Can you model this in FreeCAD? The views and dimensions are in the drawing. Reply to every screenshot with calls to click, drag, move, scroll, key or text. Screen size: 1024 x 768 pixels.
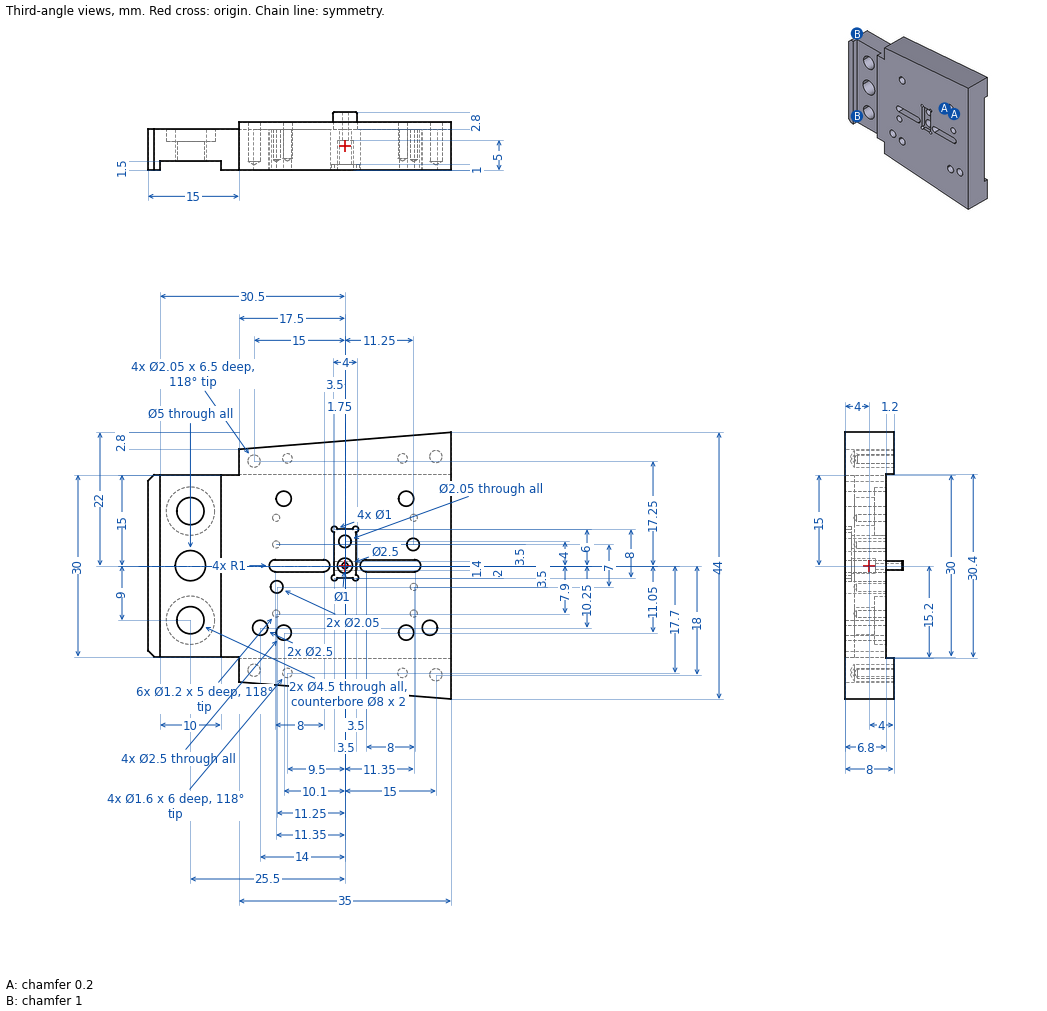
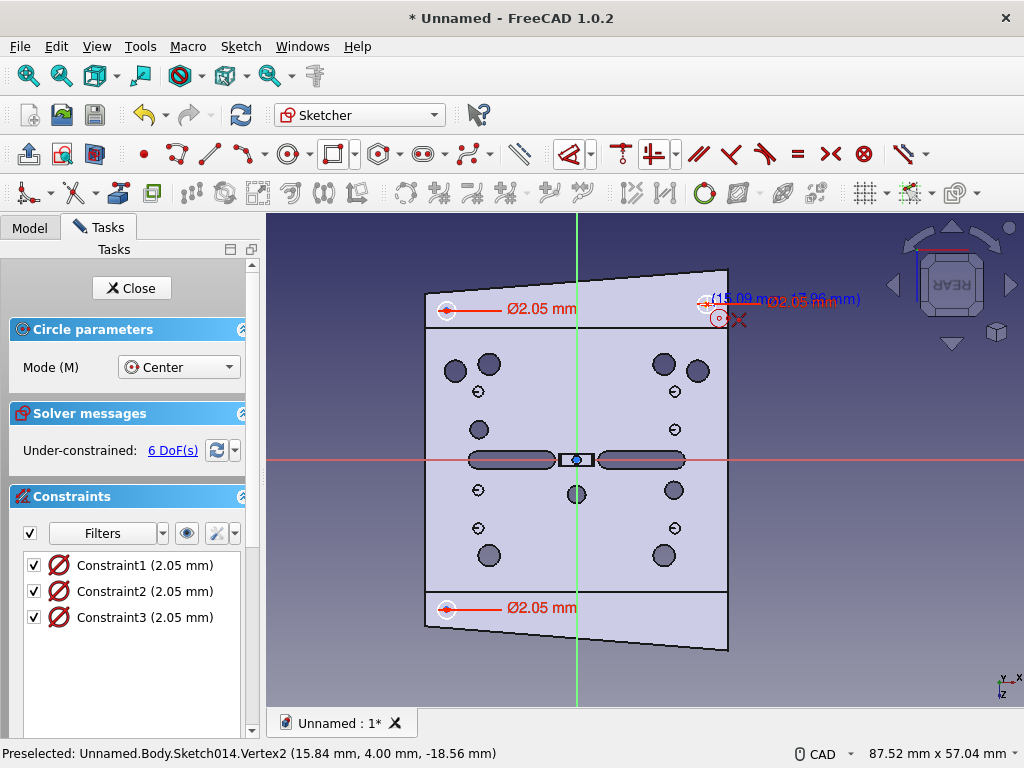
scroll(707, 616, up, 5)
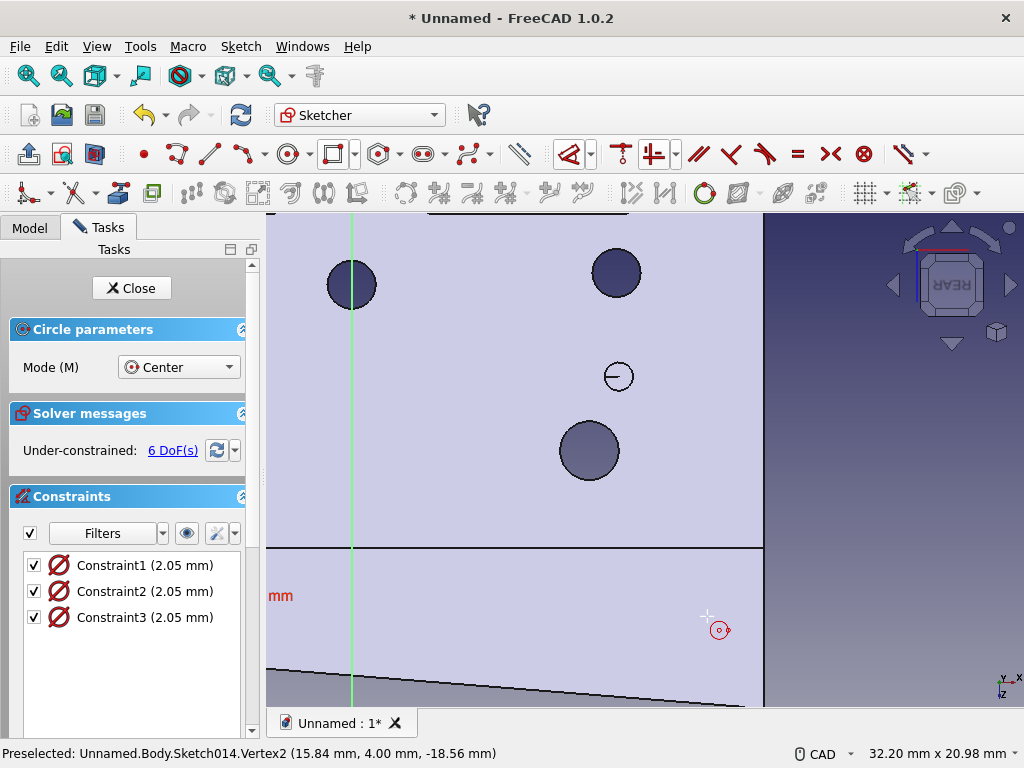
click(705, 614)
move(722, 597)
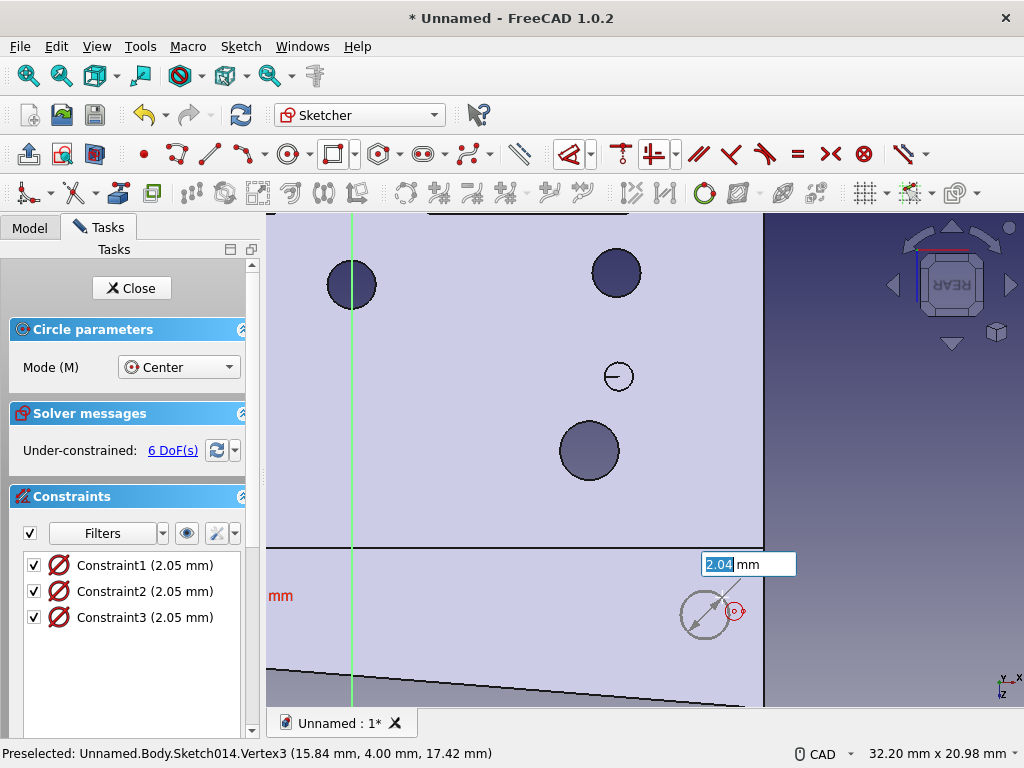
text(2.05)
key(Return)
key(Escape)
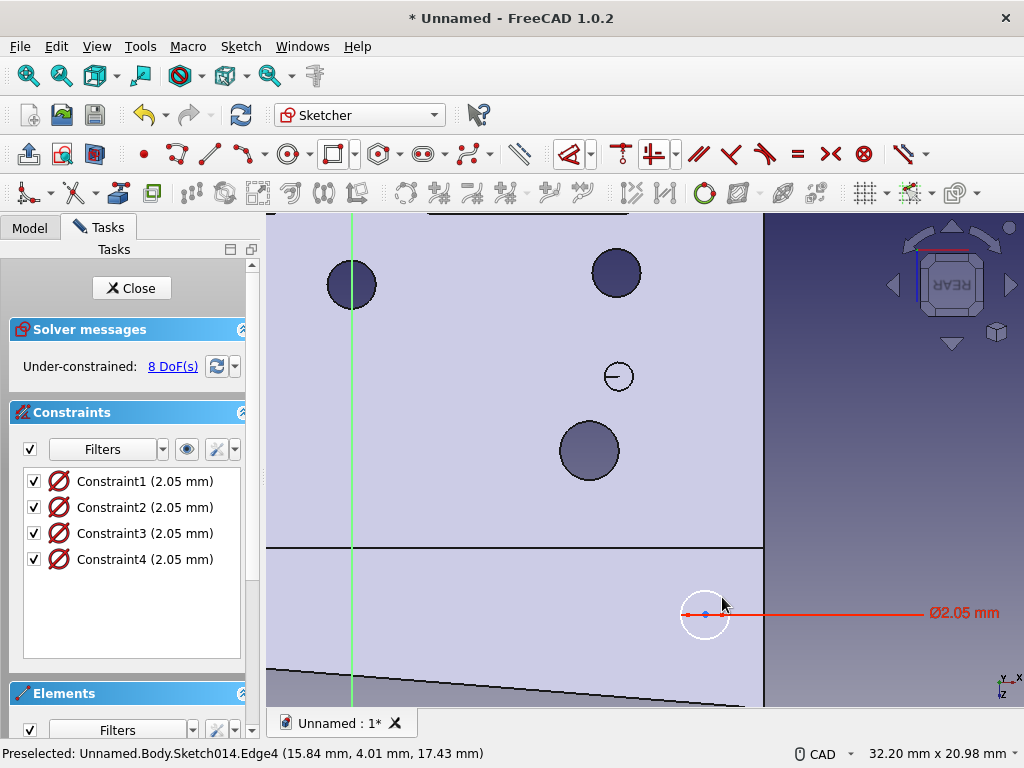
scroll(707, 617, down, 5)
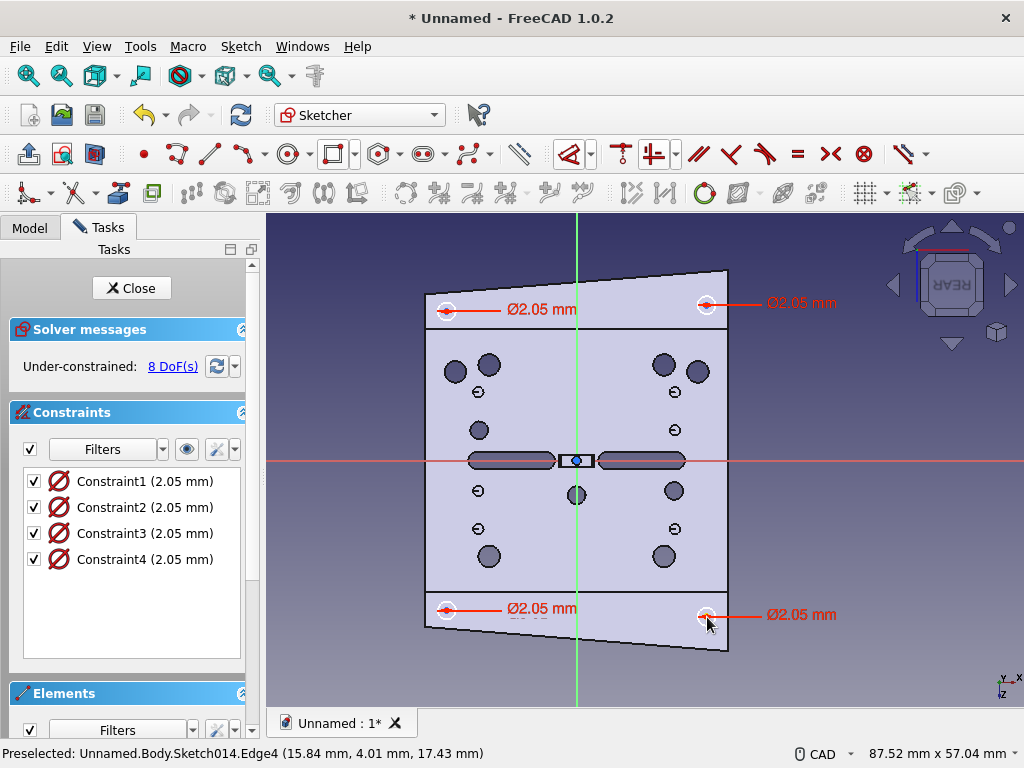
click(447, 611)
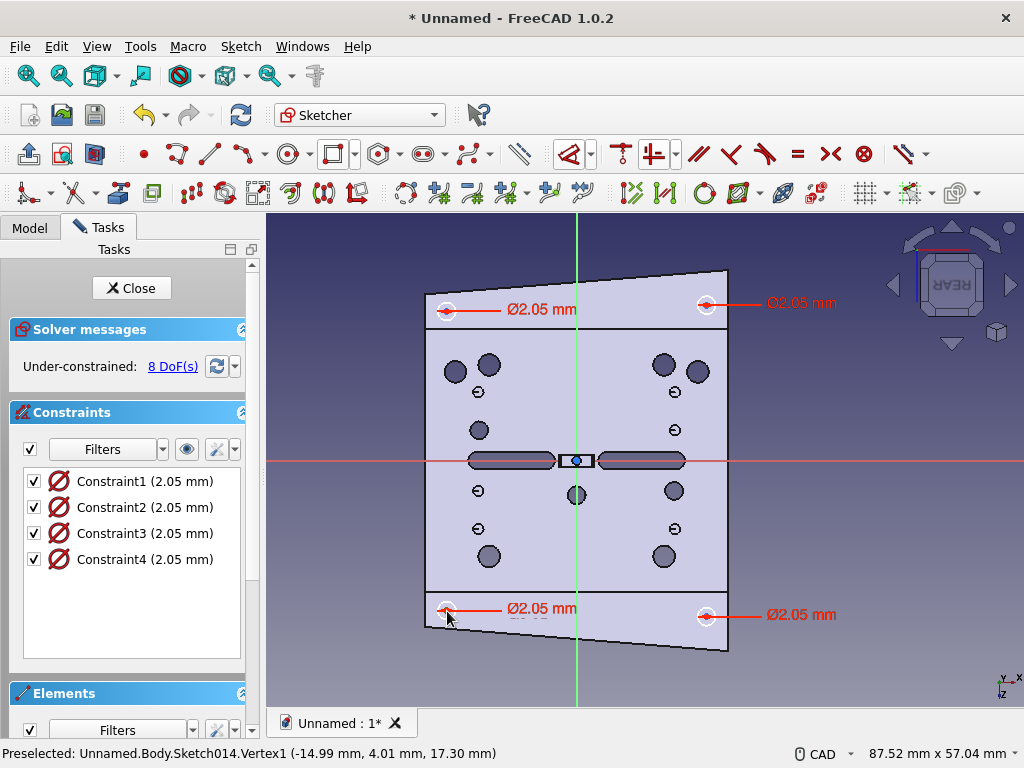
click(447, 311)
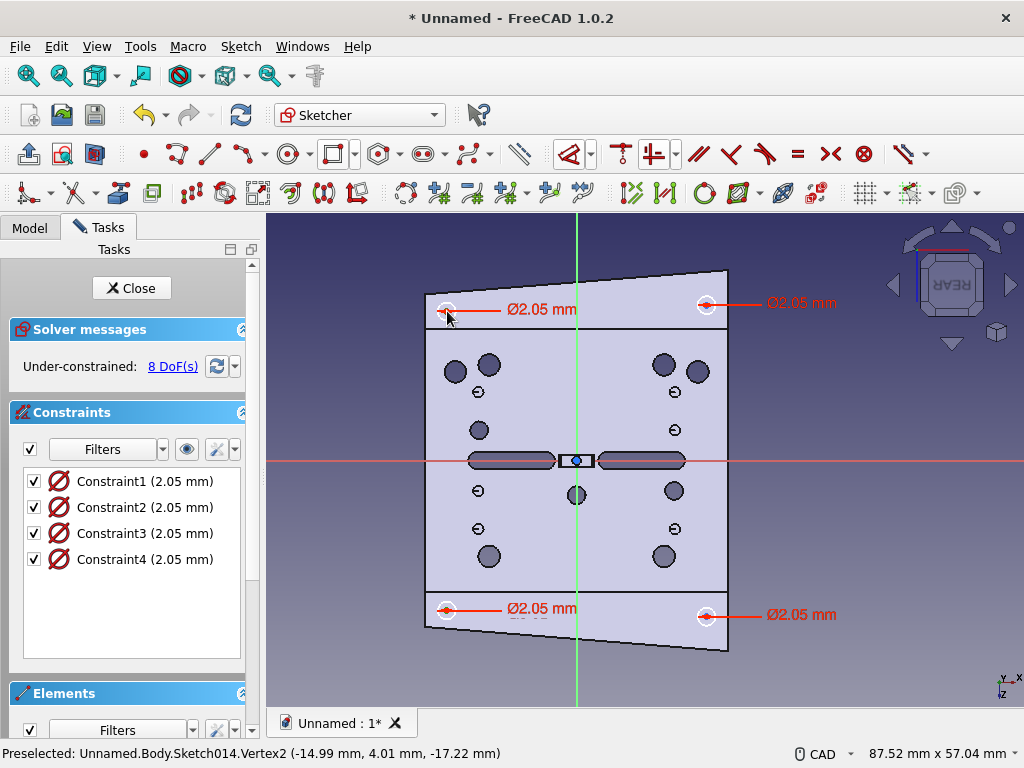
click(334, 461)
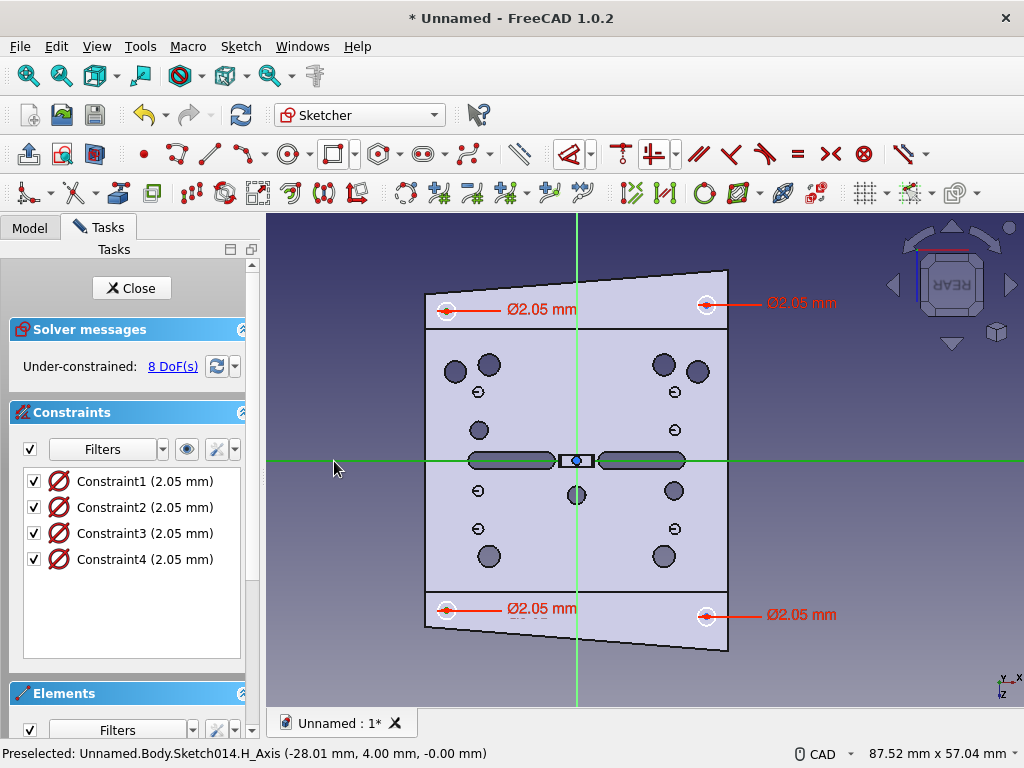
click(831, 154)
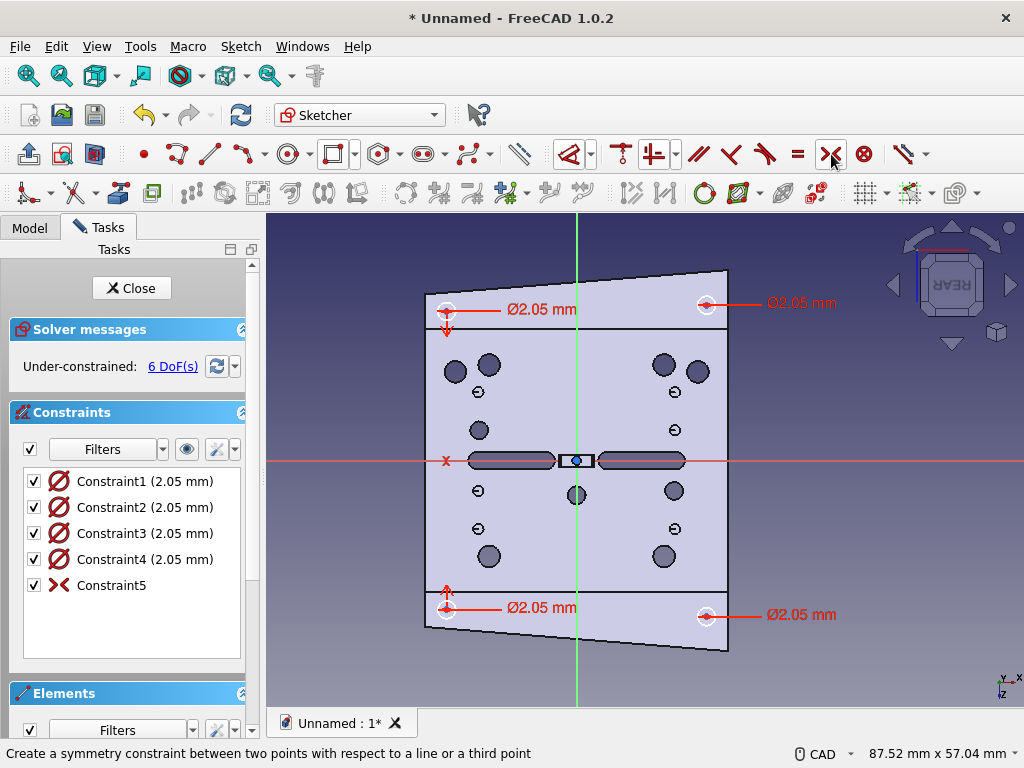
click(707, 305)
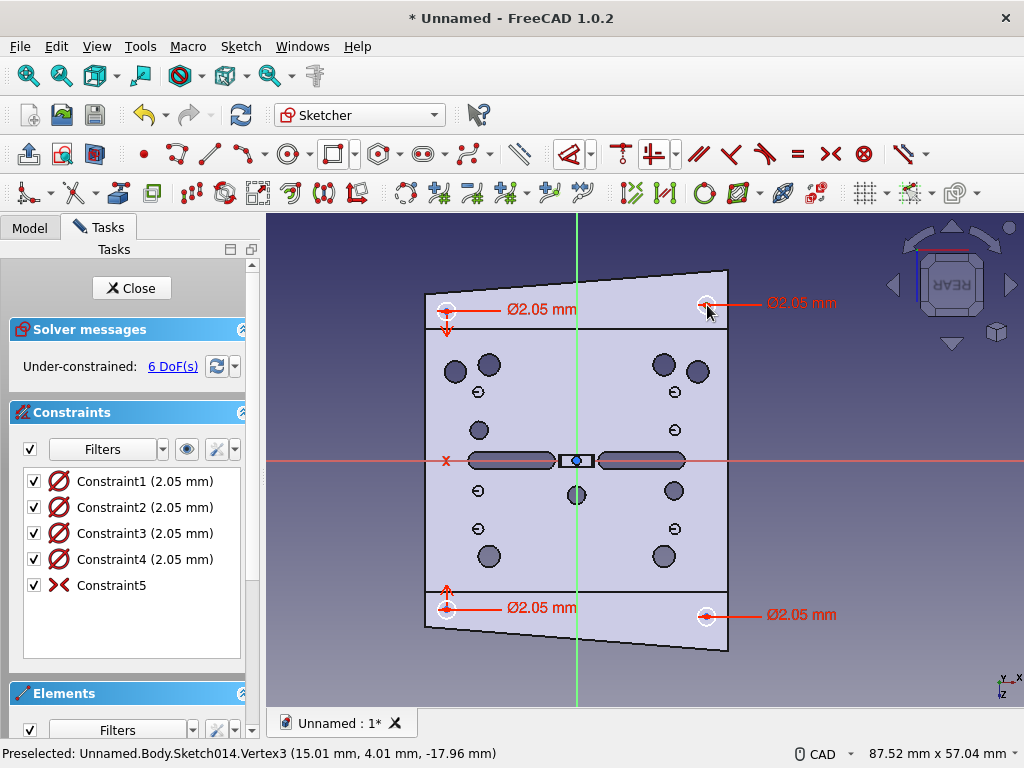
click(707, 617)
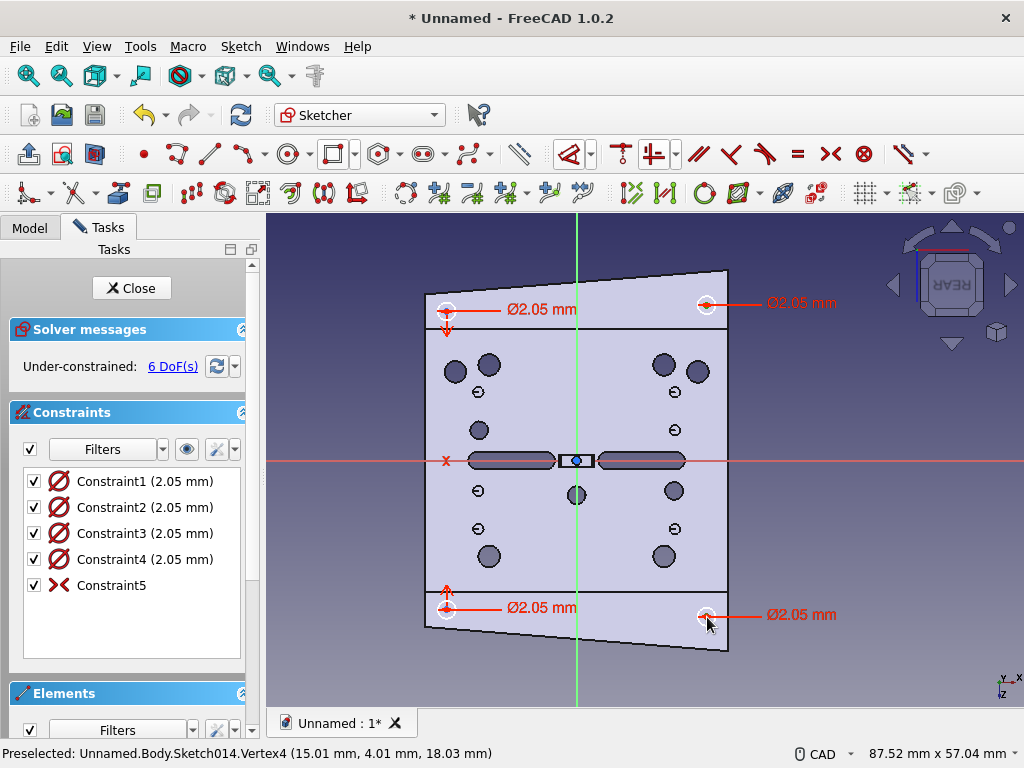
click(334, 461)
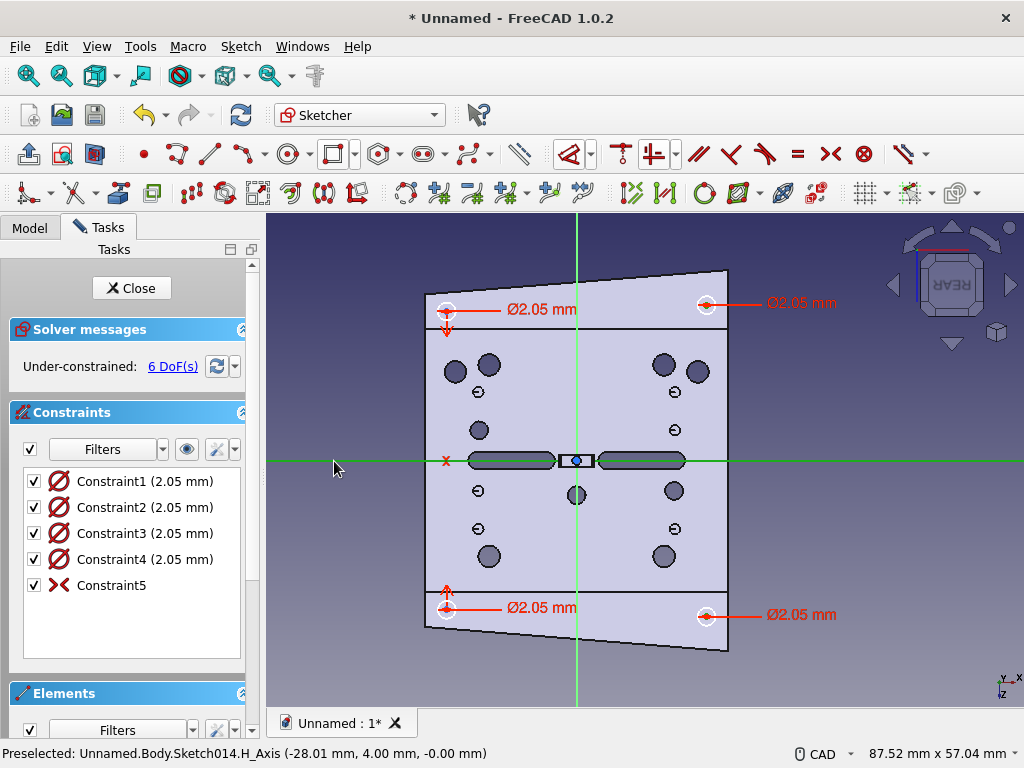
click(831, 154)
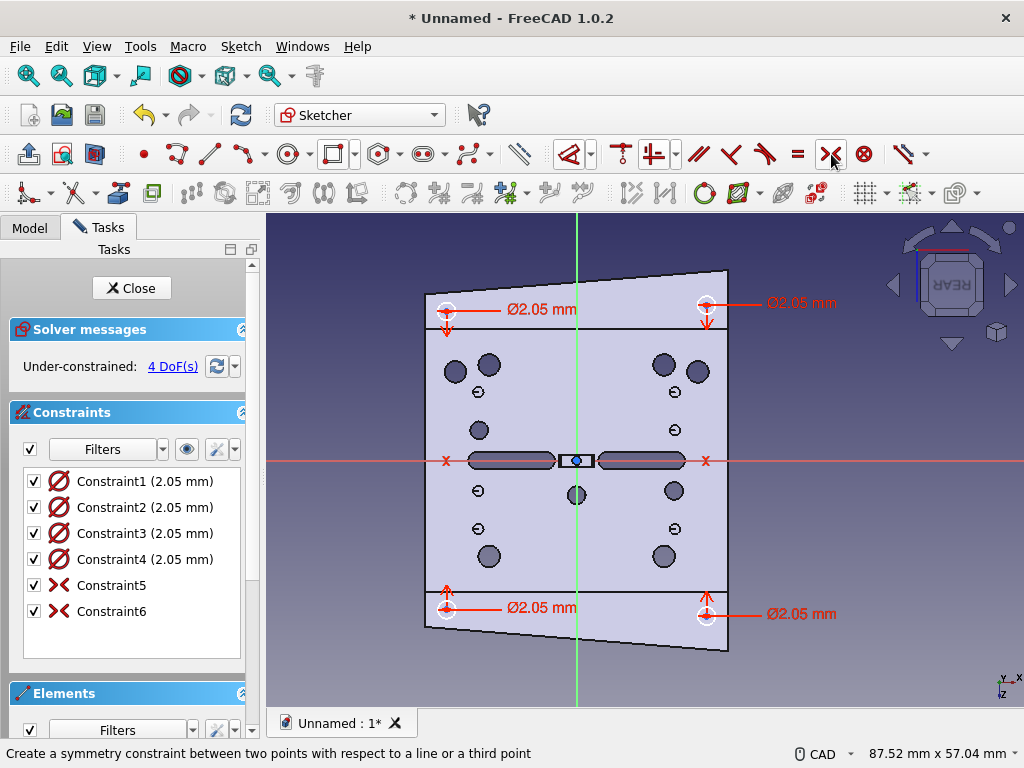
click(447, 610)